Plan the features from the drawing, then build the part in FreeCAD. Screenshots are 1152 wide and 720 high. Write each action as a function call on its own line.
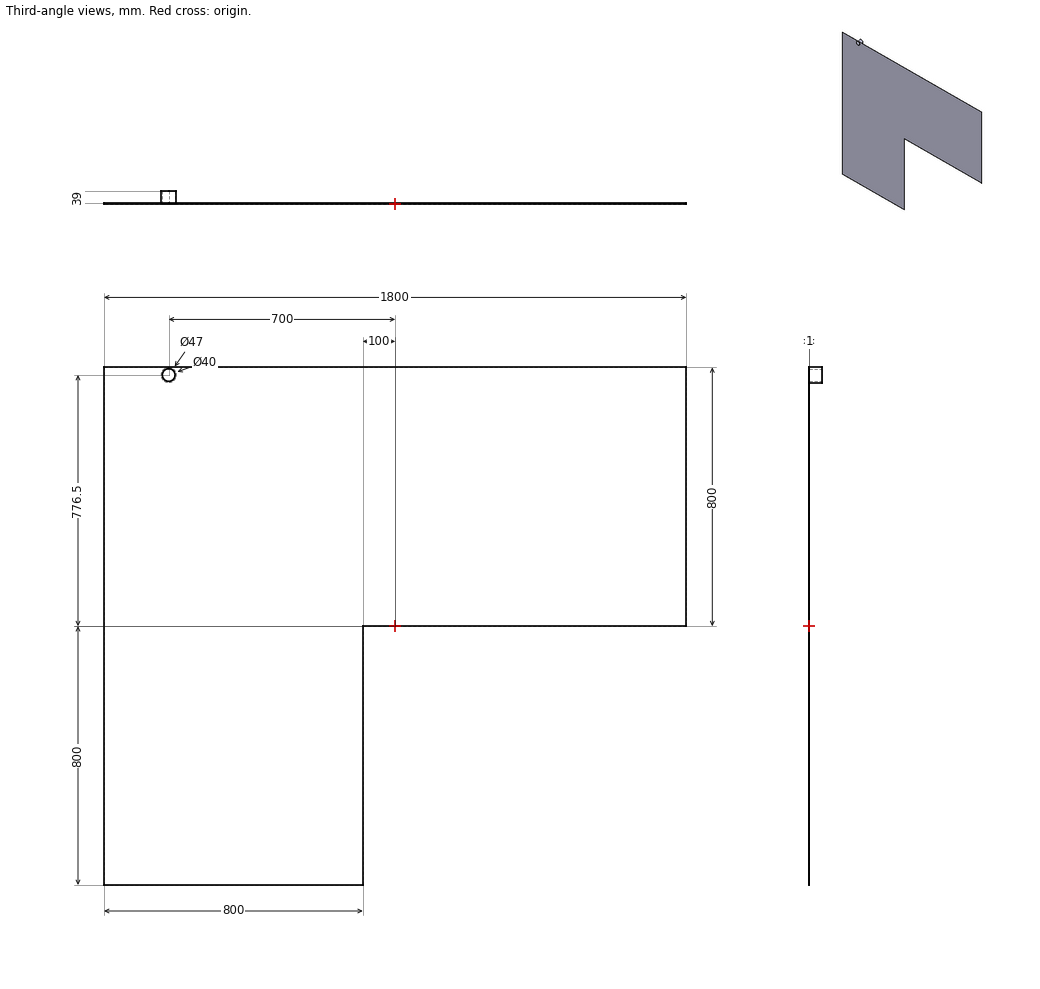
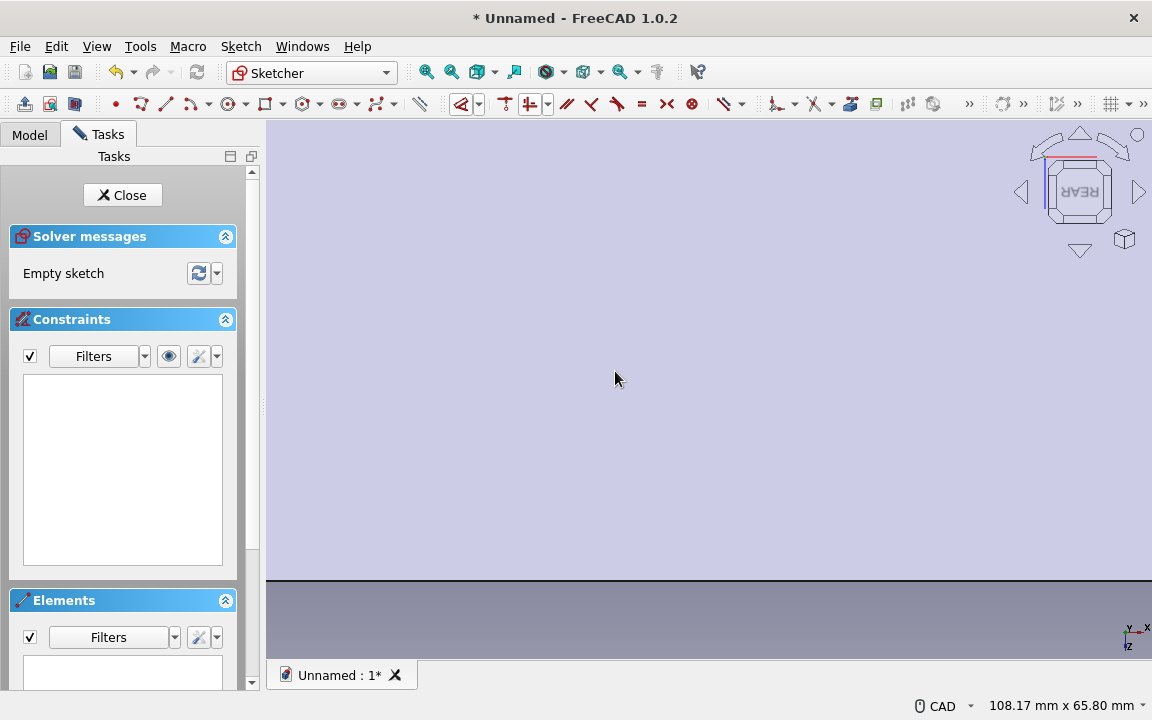
click(228, 104)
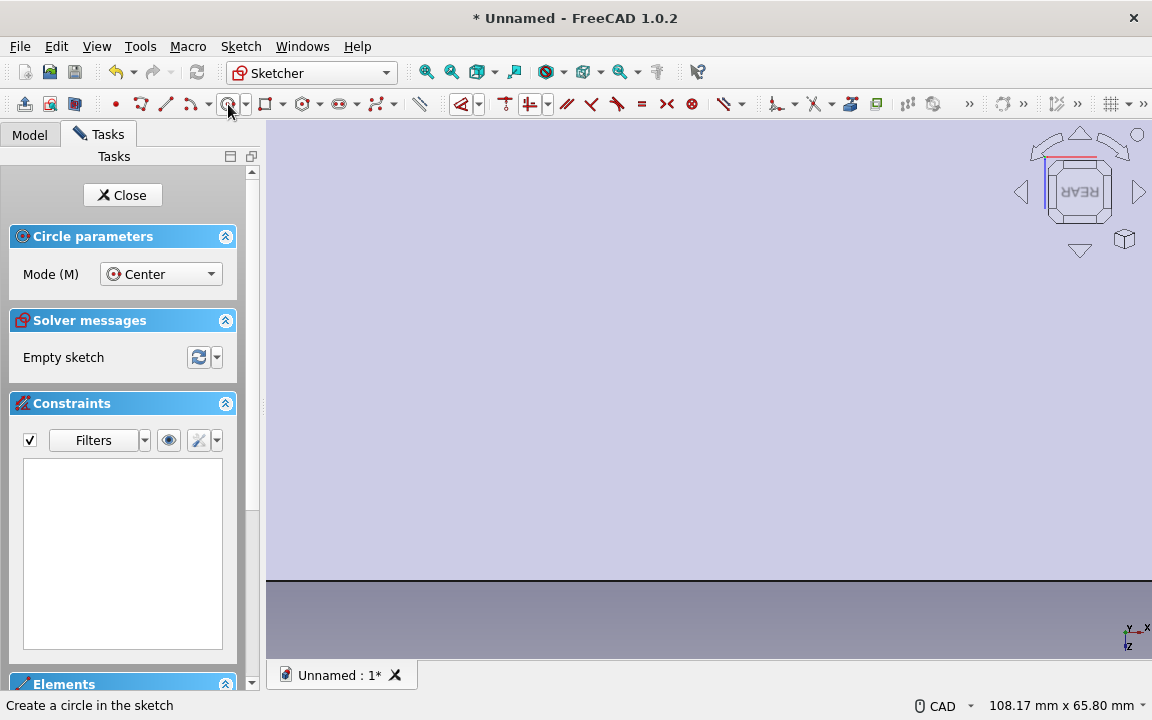
click(640, 389)
click(756, 273)
key(Escape)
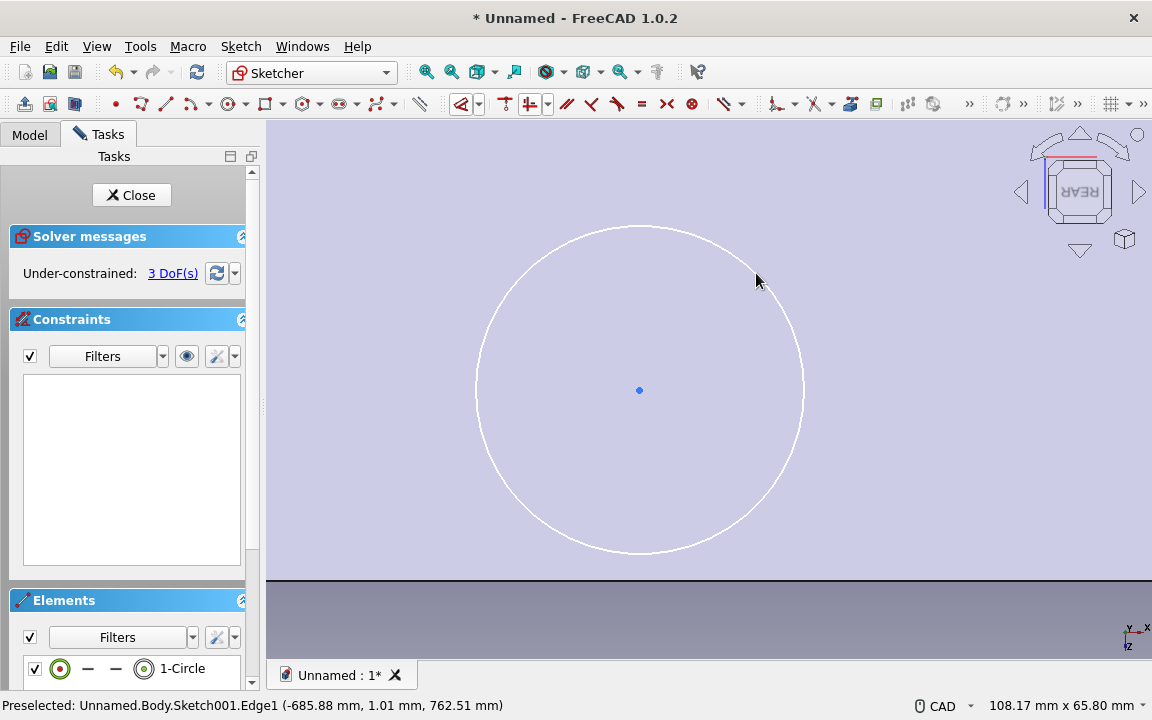
click(756, 274)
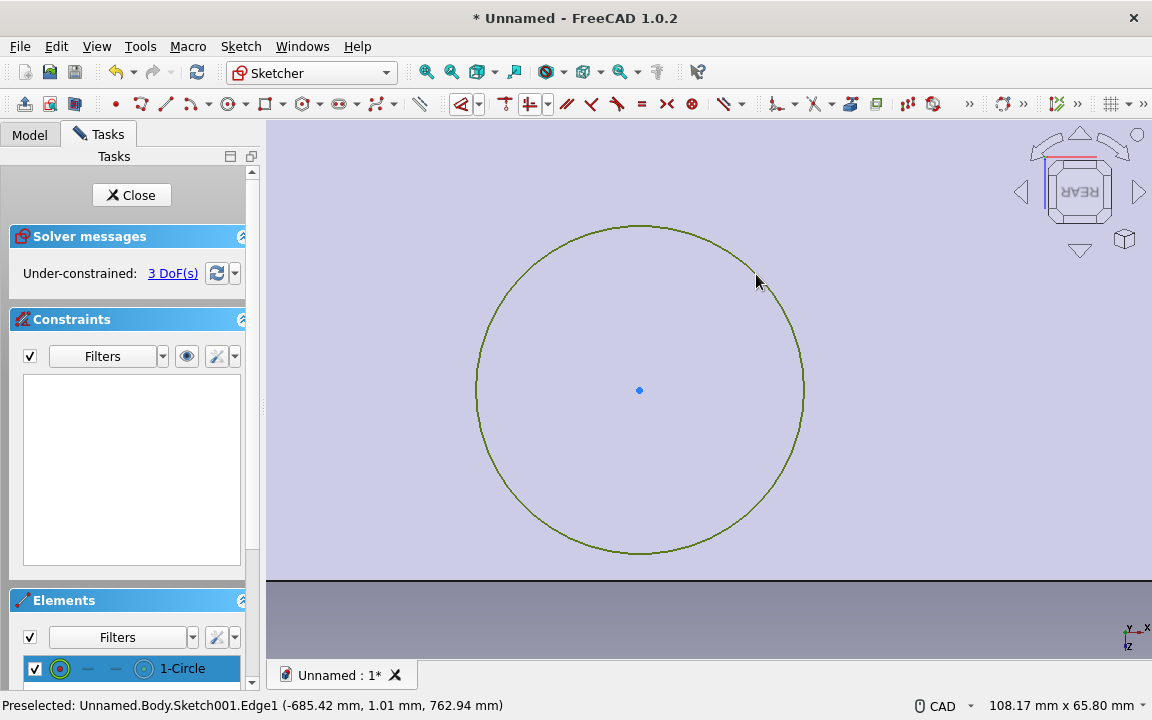
key(k)
key(o)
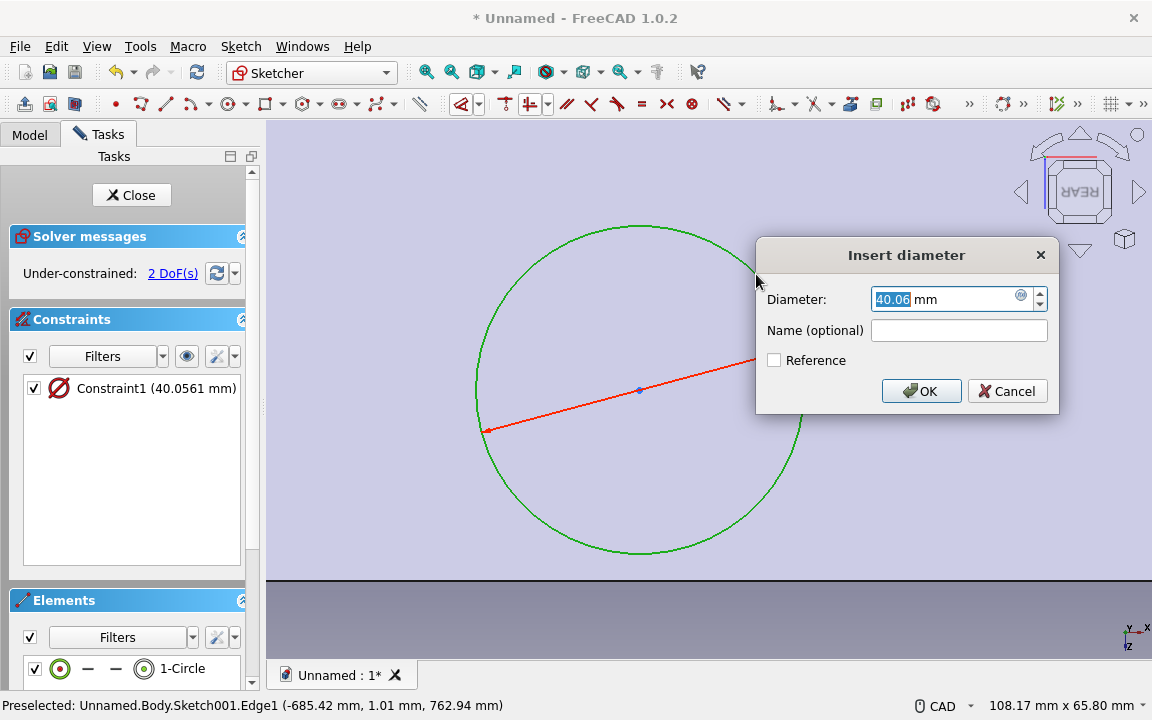
text(40)
key(Return)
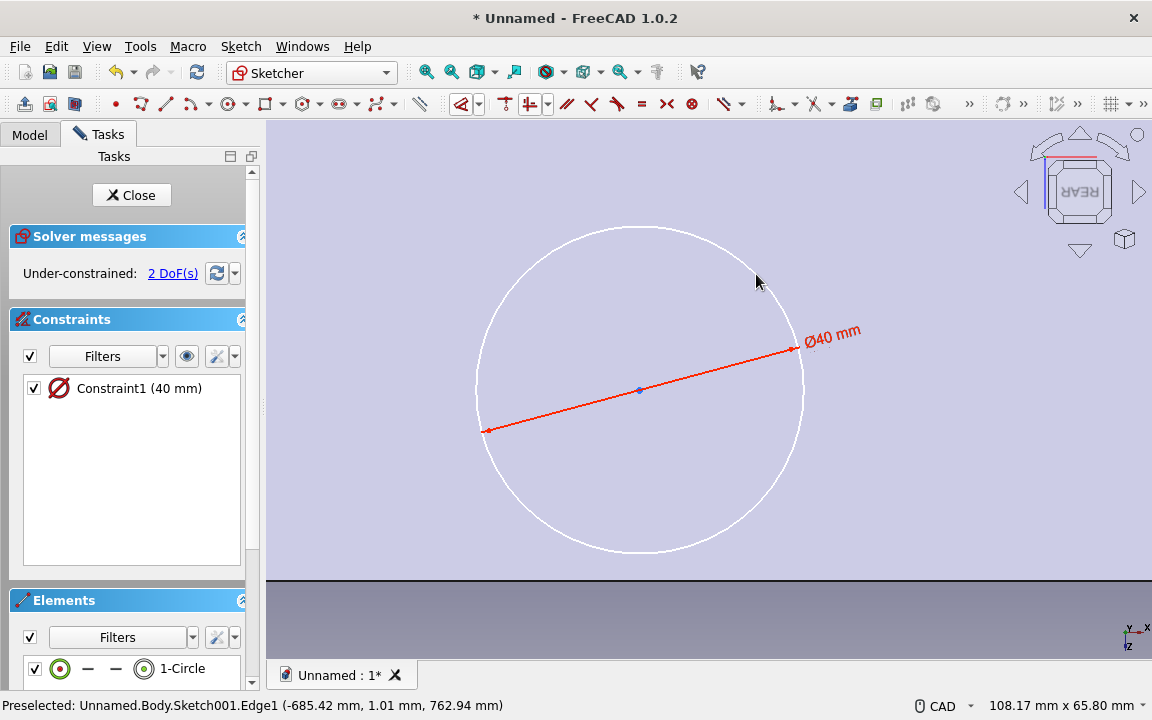
click(640, 390)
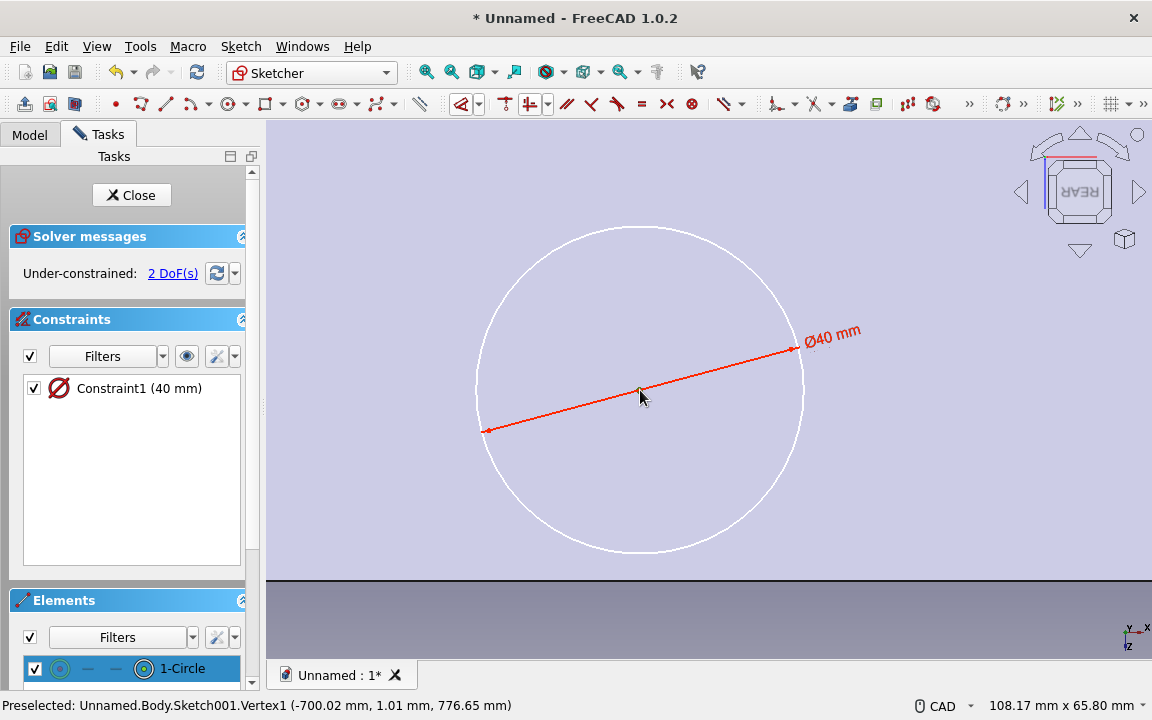
click(478, 104)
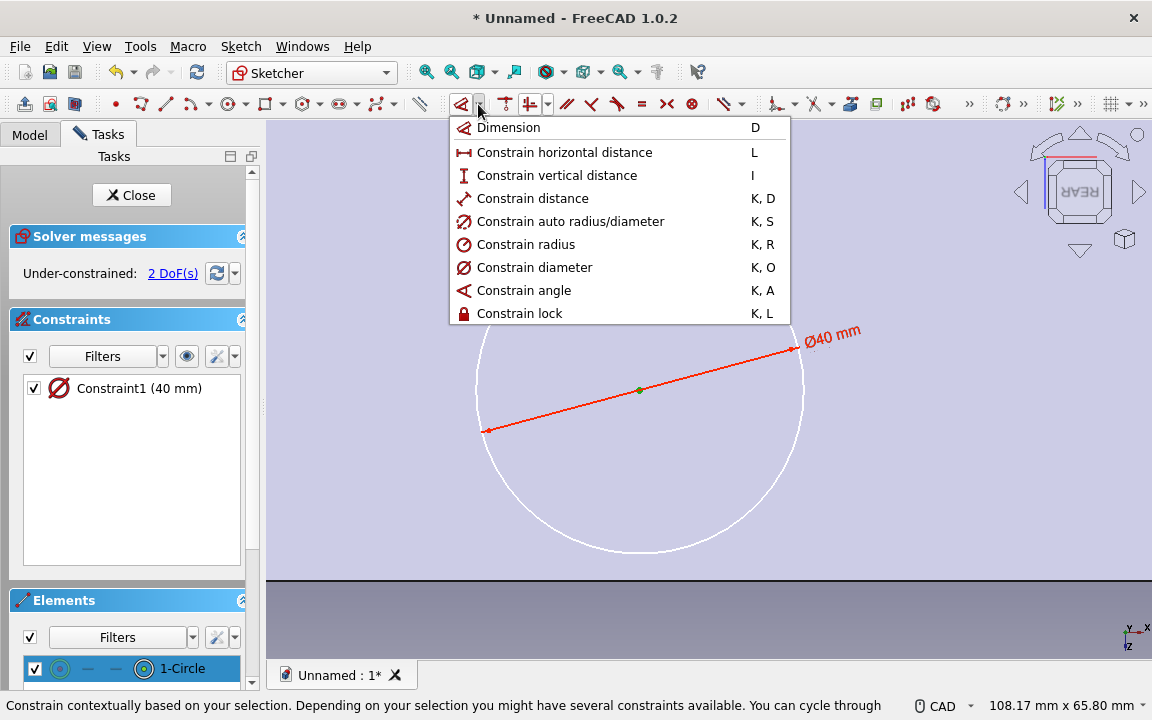
click(620, 152)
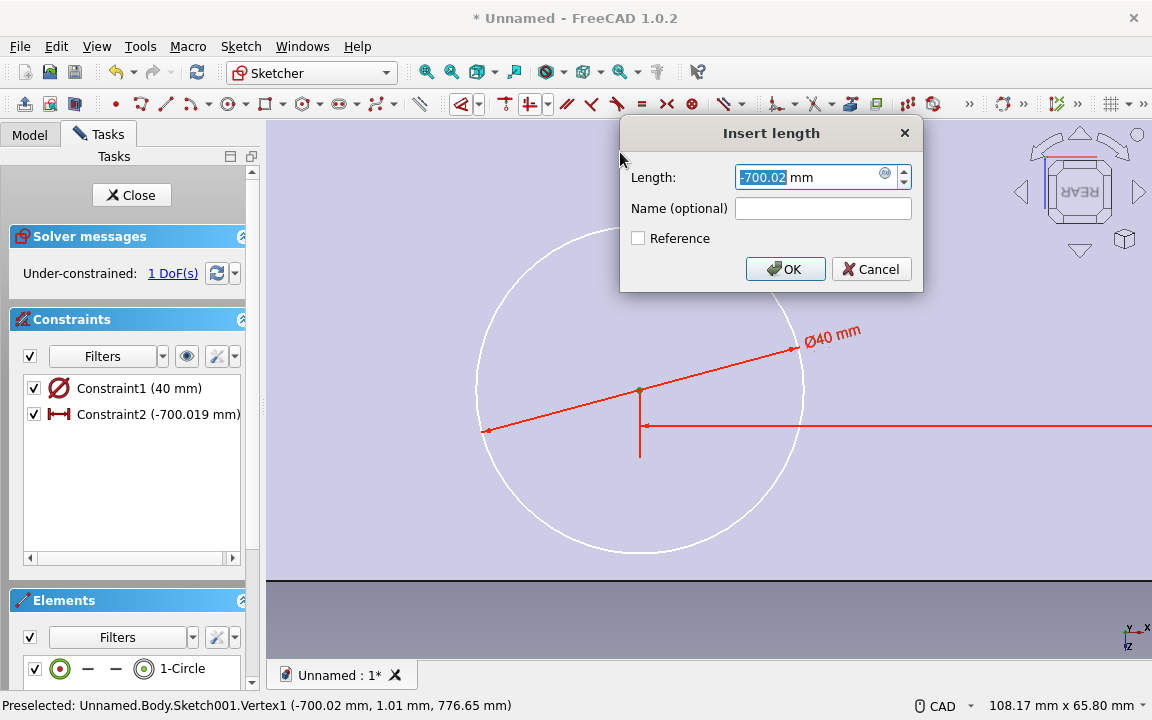
text(-700)
key(Return)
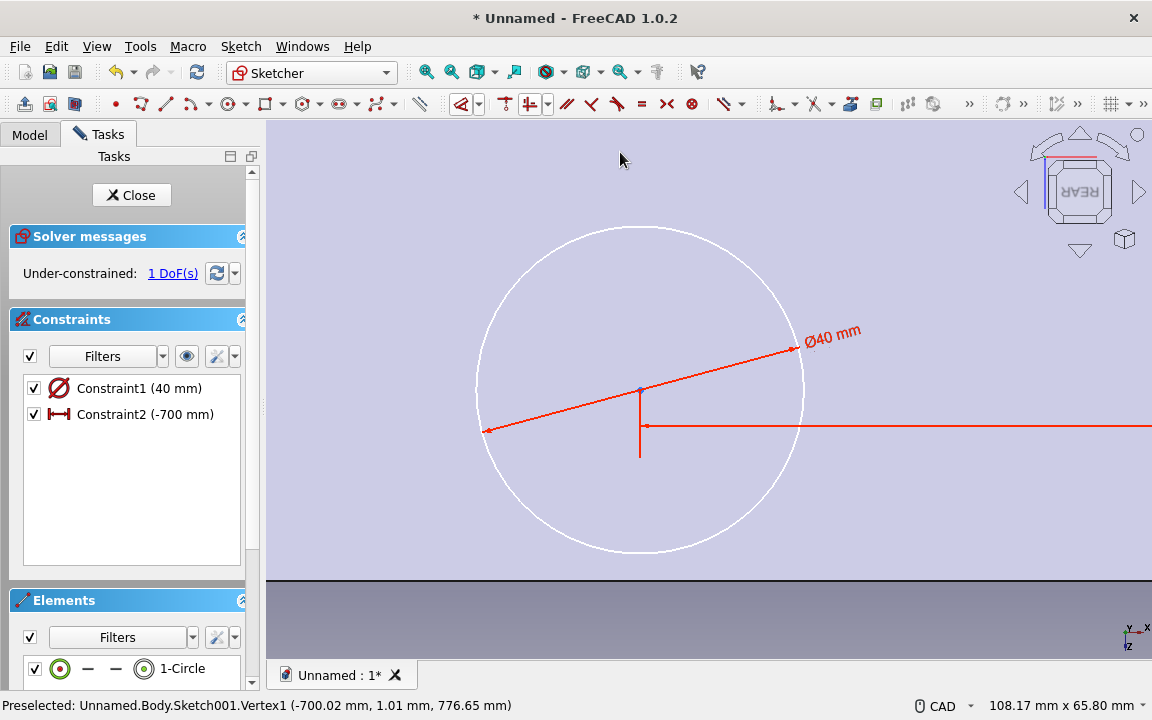
click(640, 390)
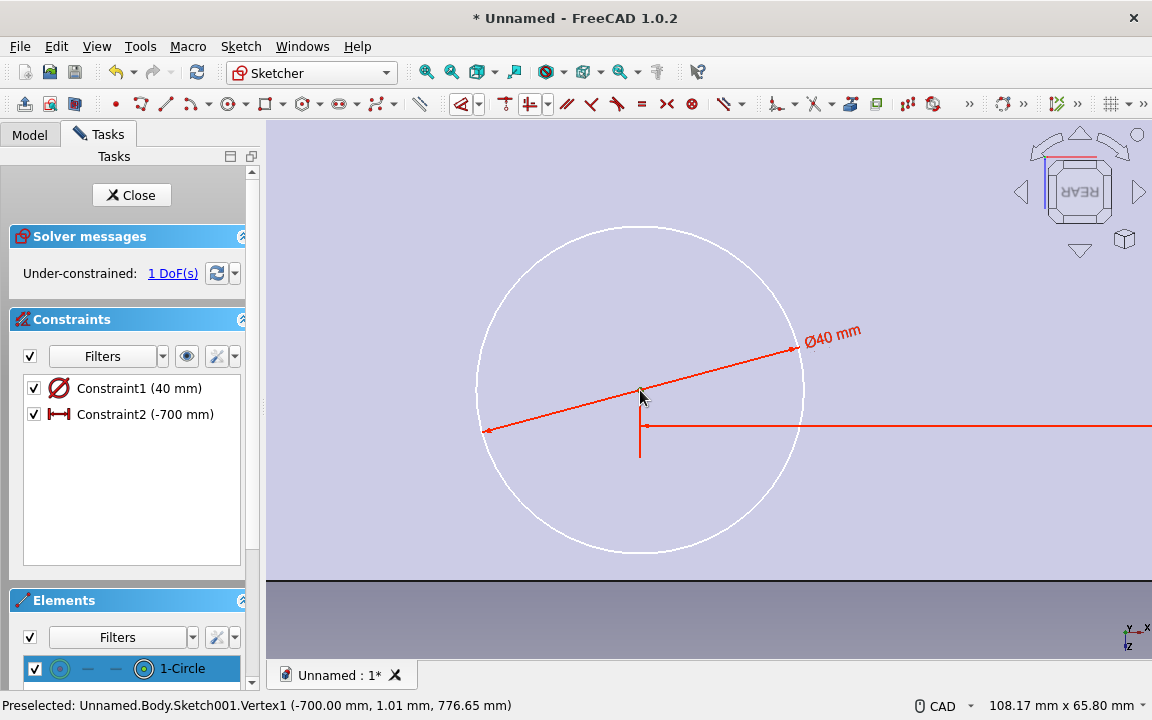
click(478, 104)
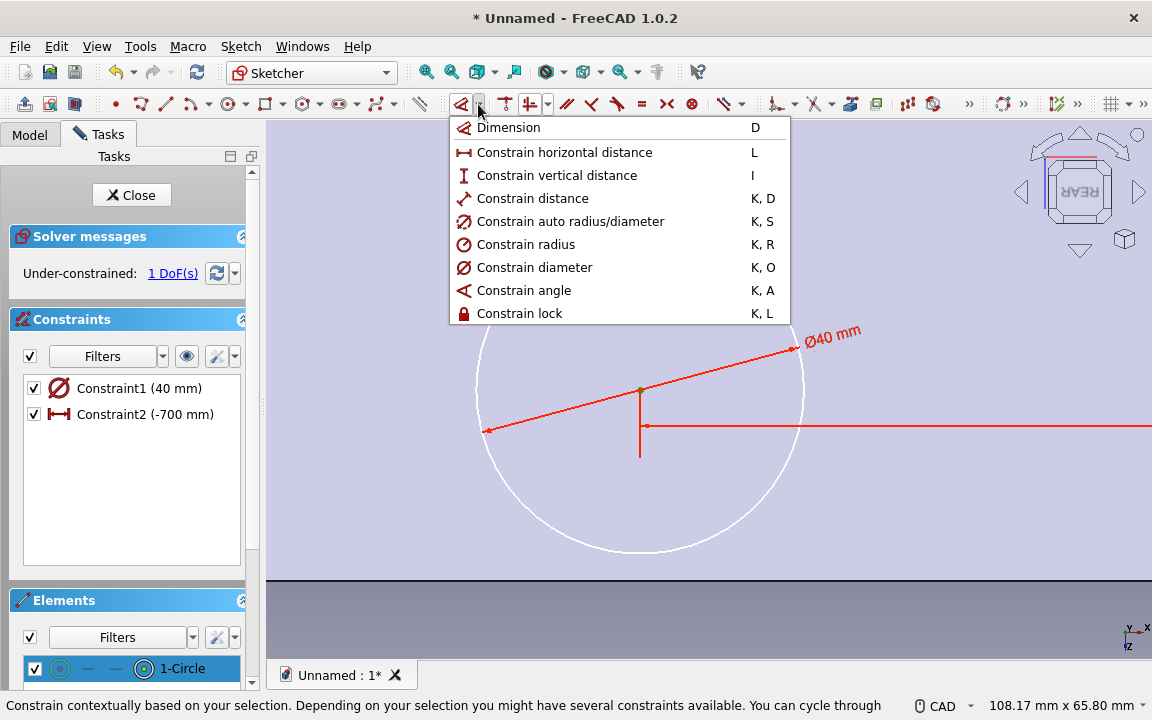
click(620, 176)